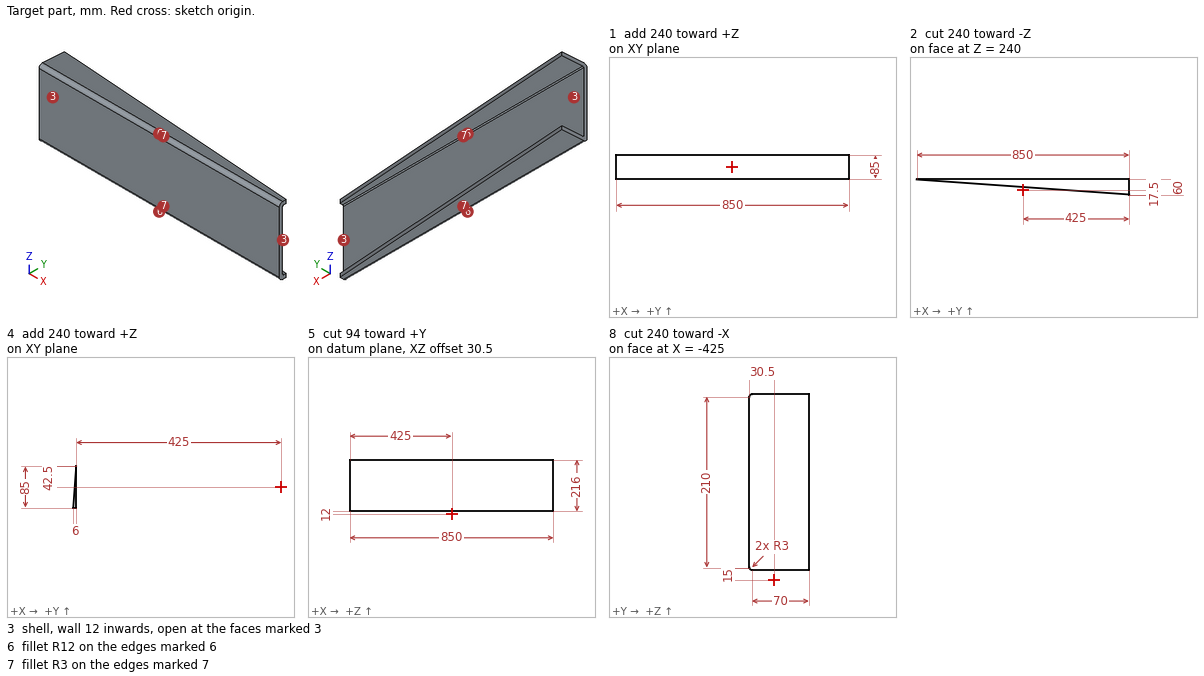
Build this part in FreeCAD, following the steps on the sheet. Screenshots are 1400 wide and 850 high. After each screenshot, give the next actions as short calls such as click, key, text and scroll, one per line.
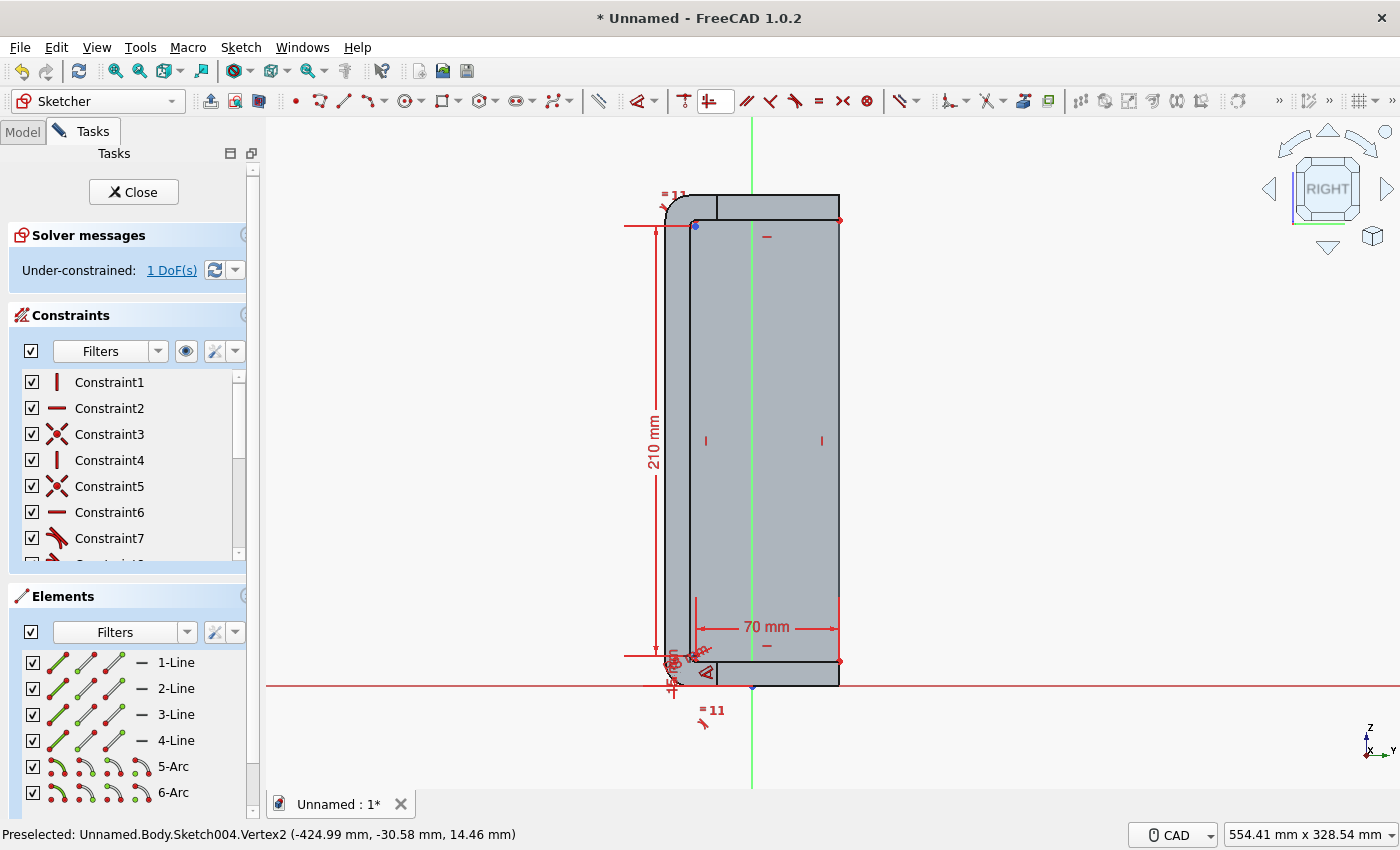
scroll(690, 226, up, 4)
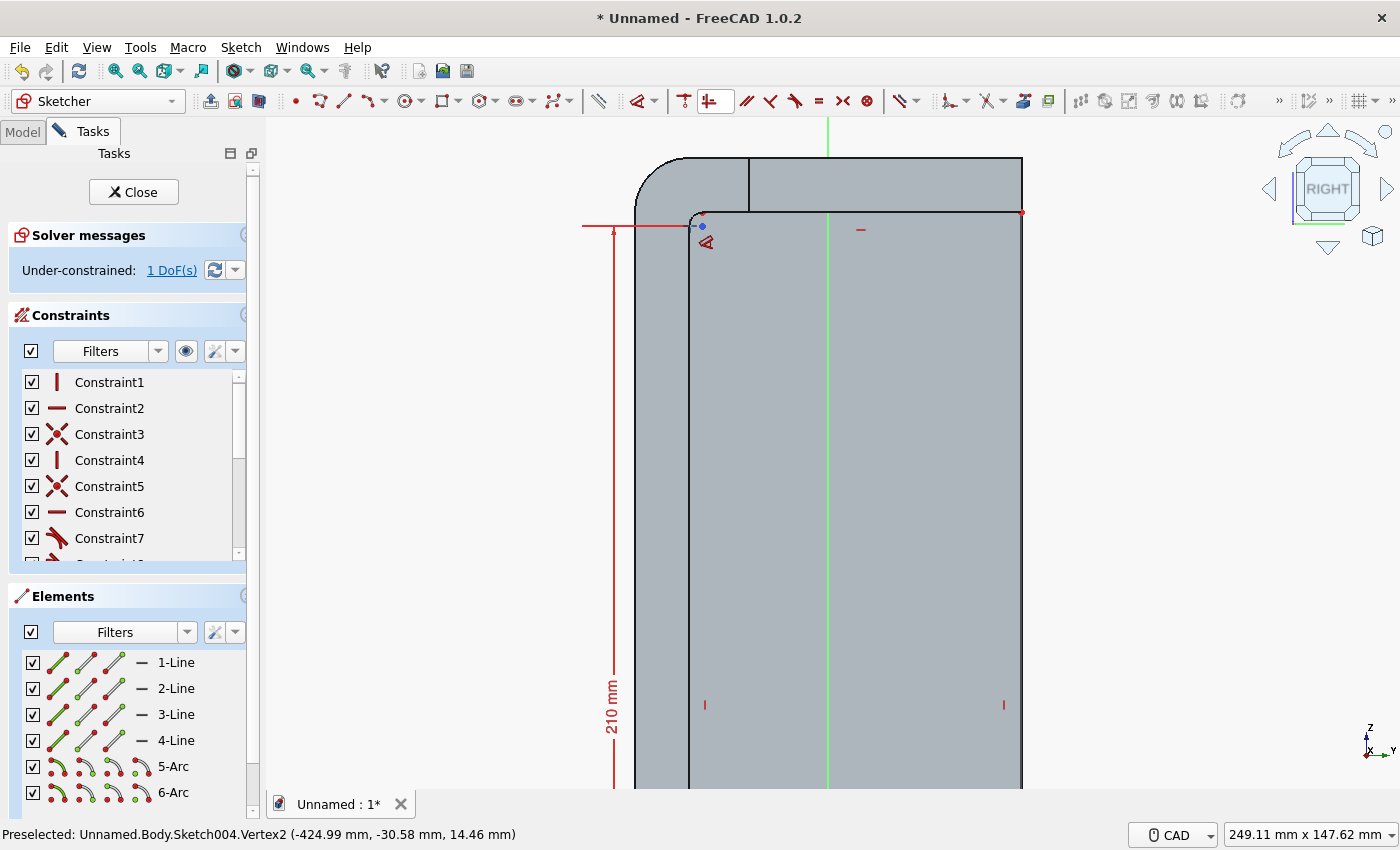
click(689, 226)
click(759, 192)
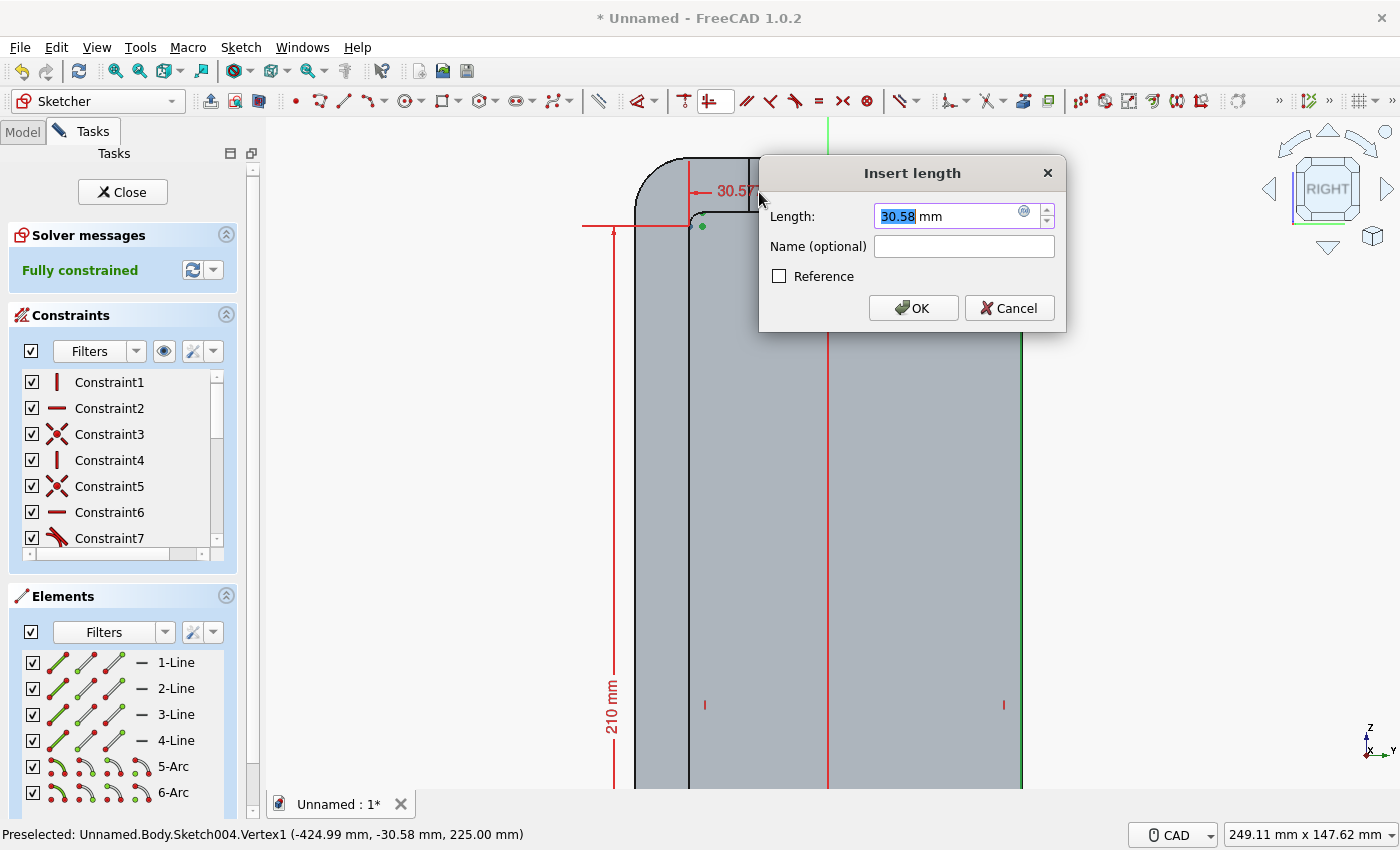
text(30.5)
key(Return)
key(Escape)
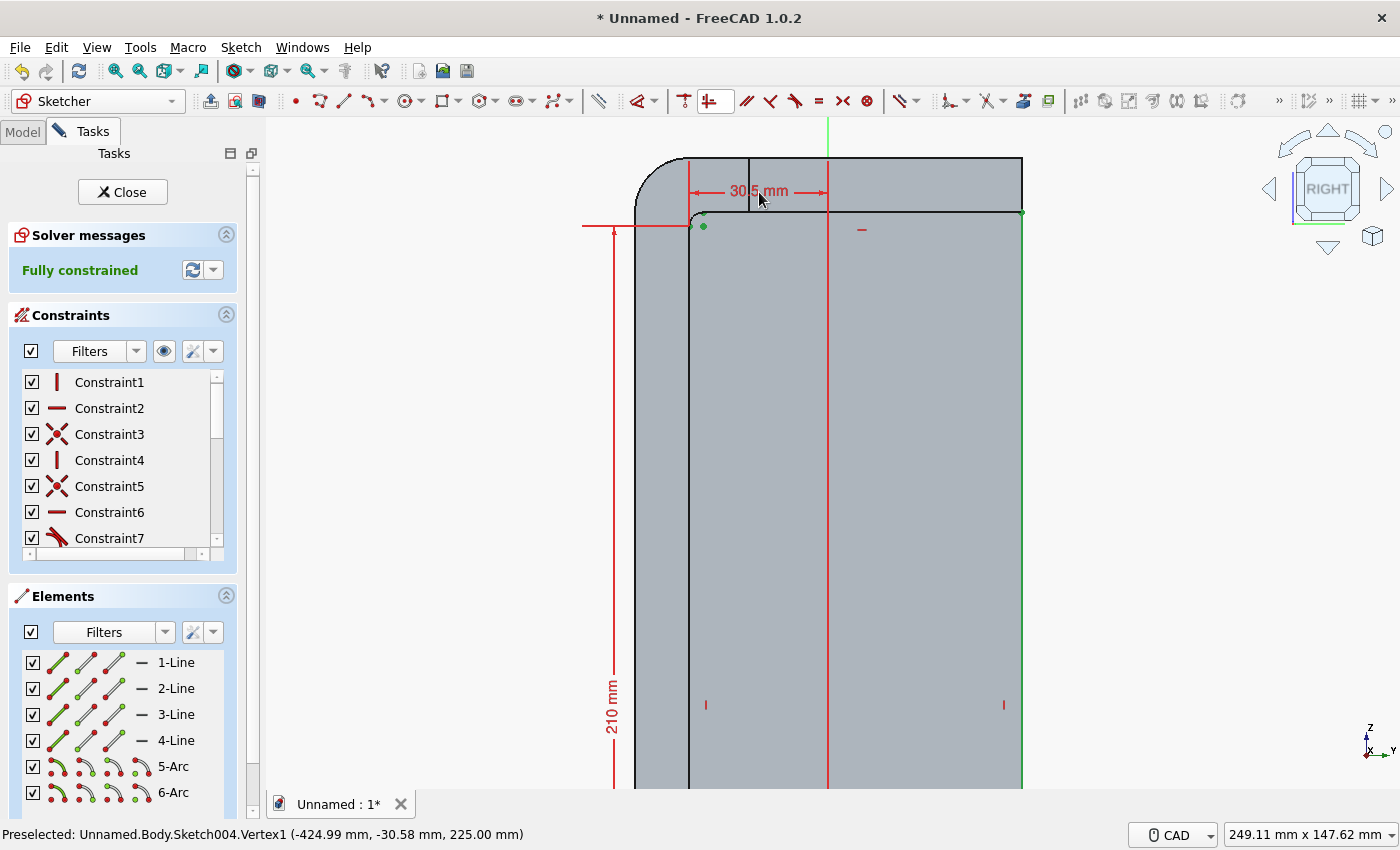
click(123, 192)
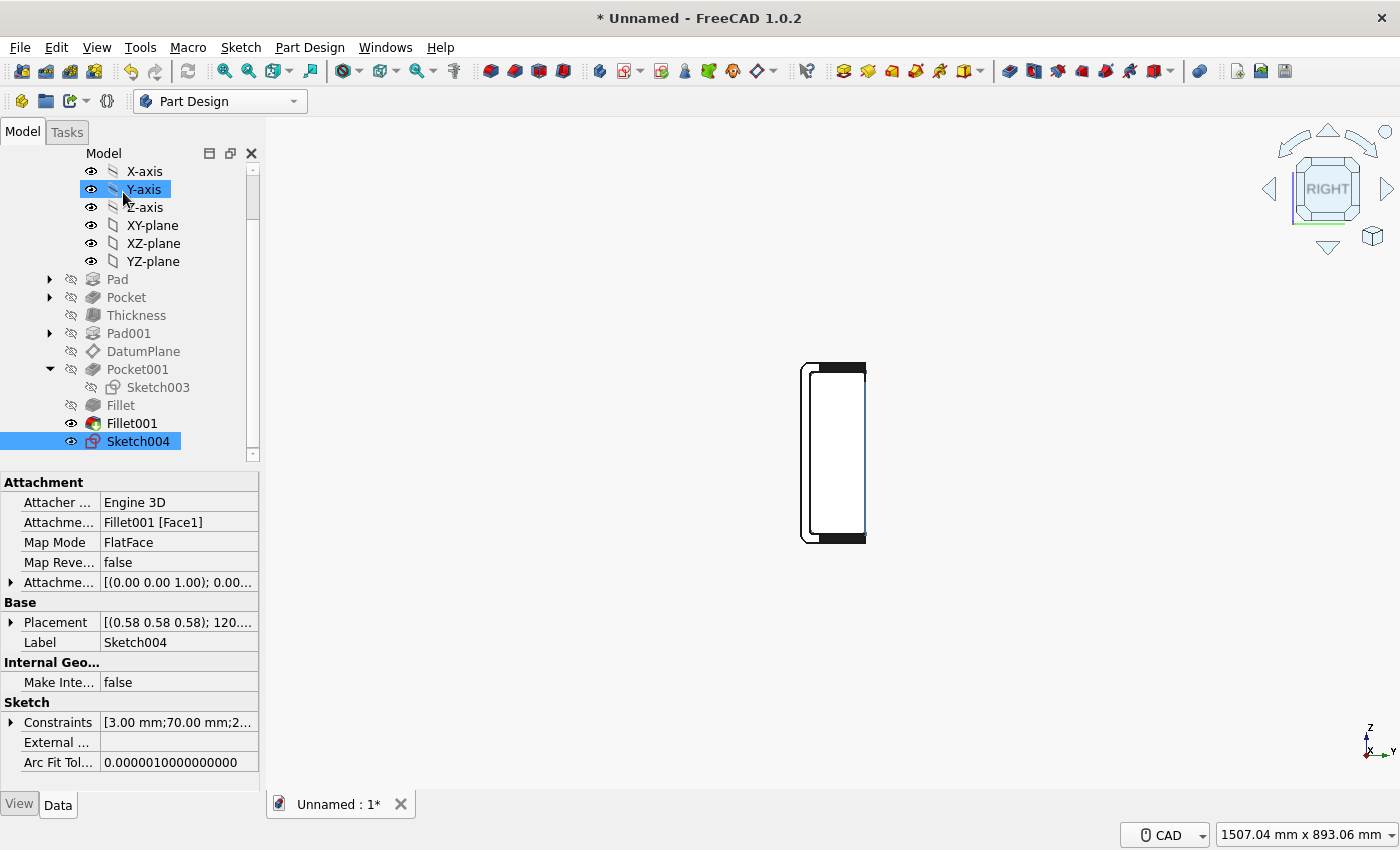
click(1010, 72)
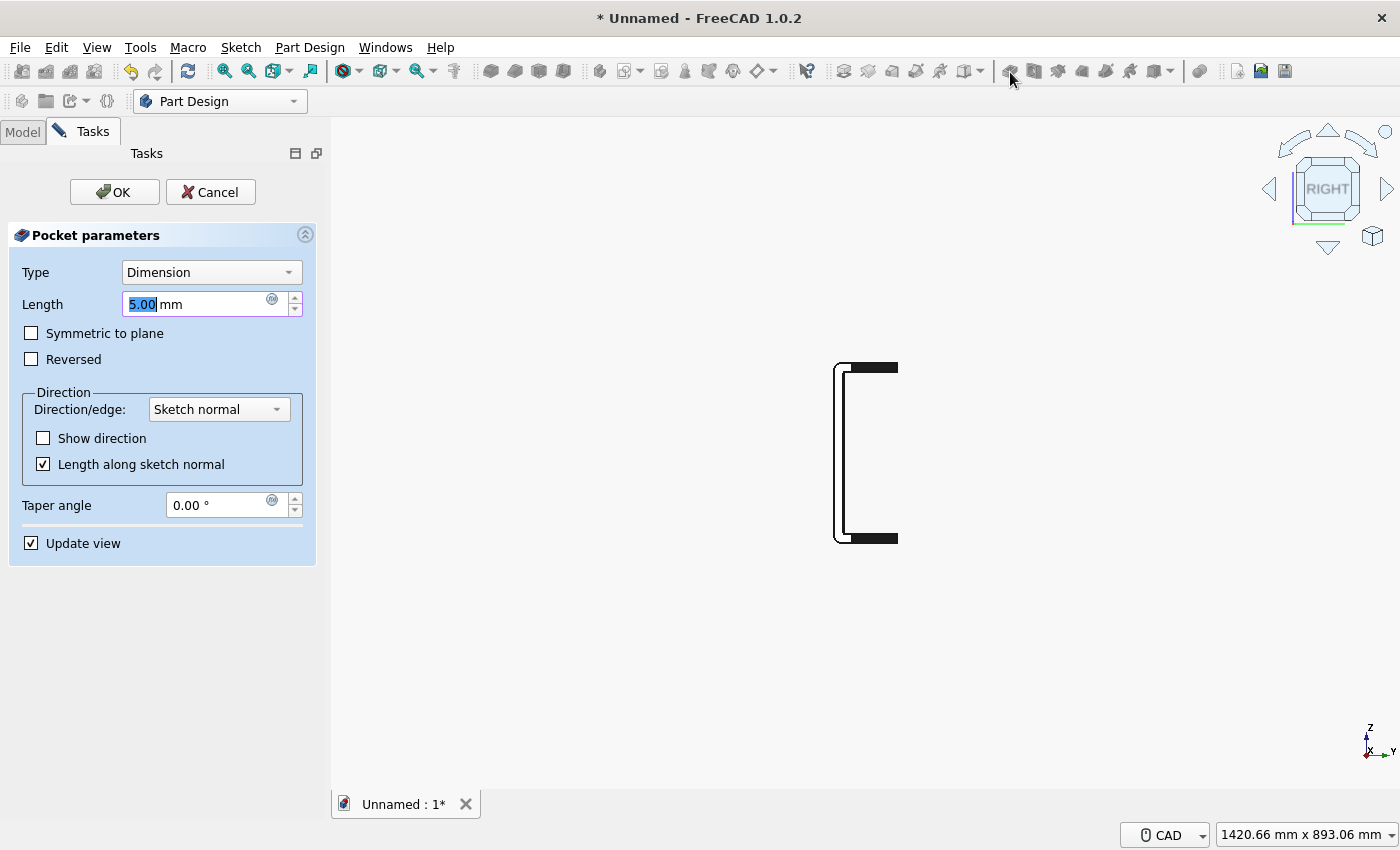
text(240)
key(Tab)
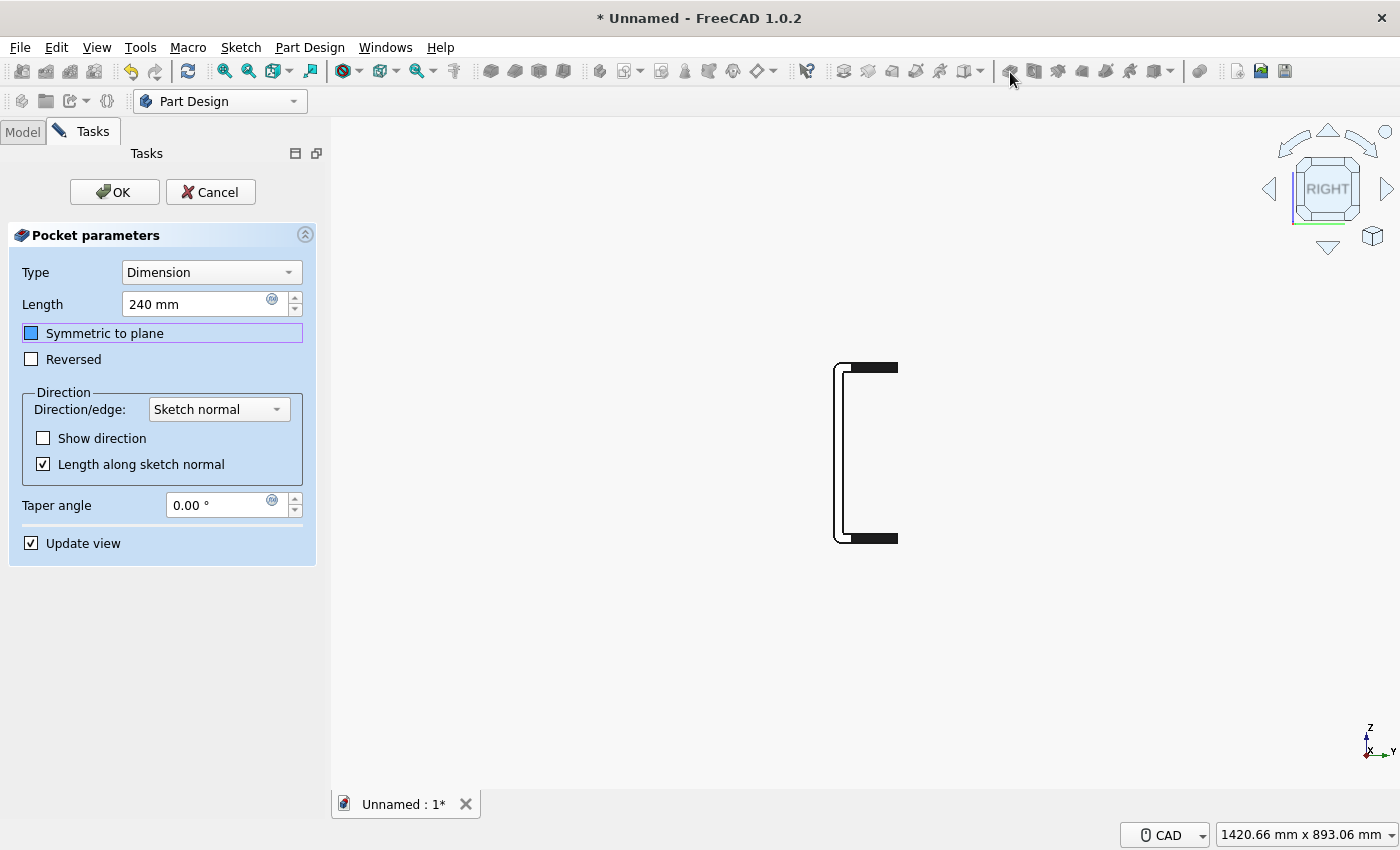
click(115, 192)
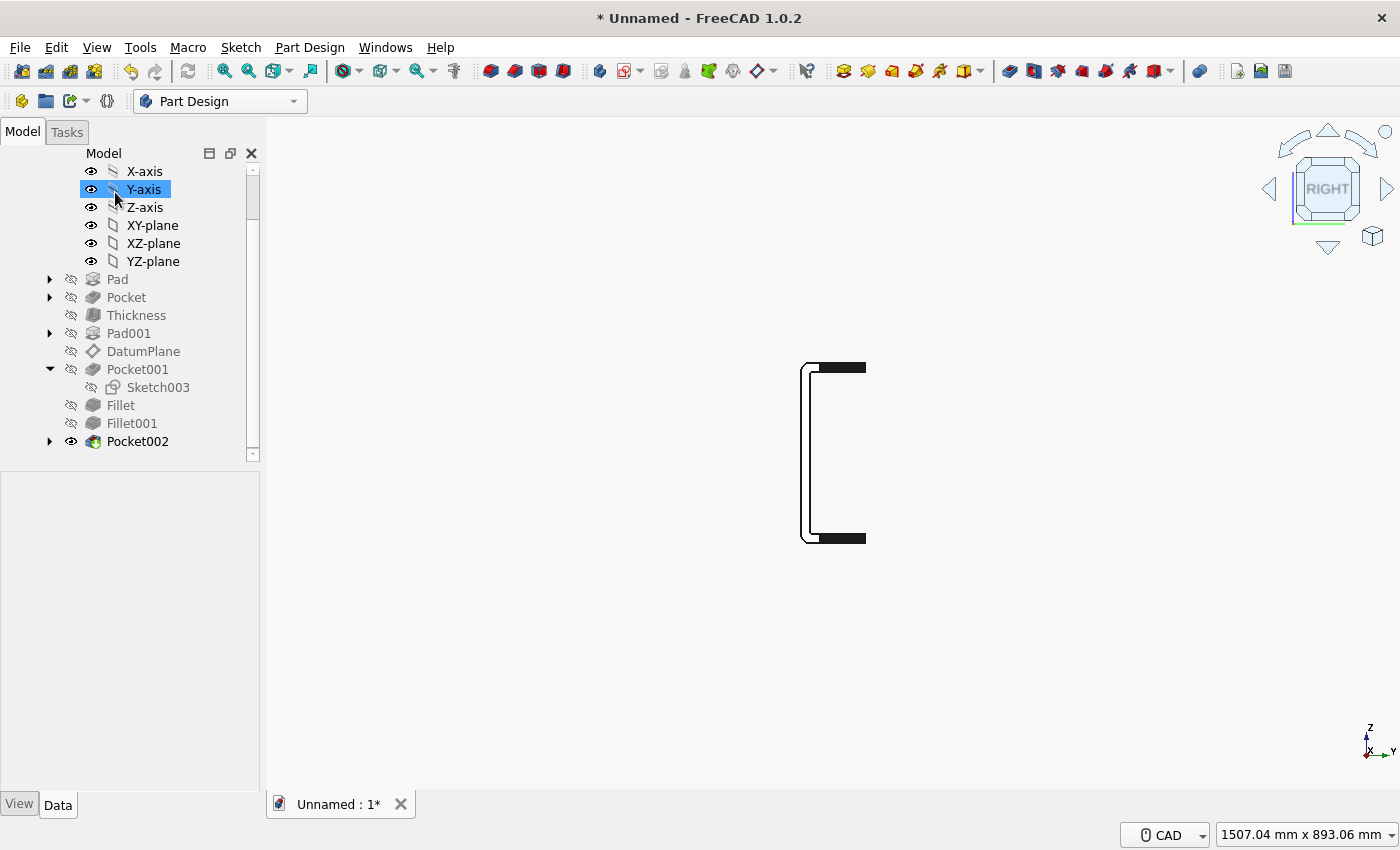
key(0)